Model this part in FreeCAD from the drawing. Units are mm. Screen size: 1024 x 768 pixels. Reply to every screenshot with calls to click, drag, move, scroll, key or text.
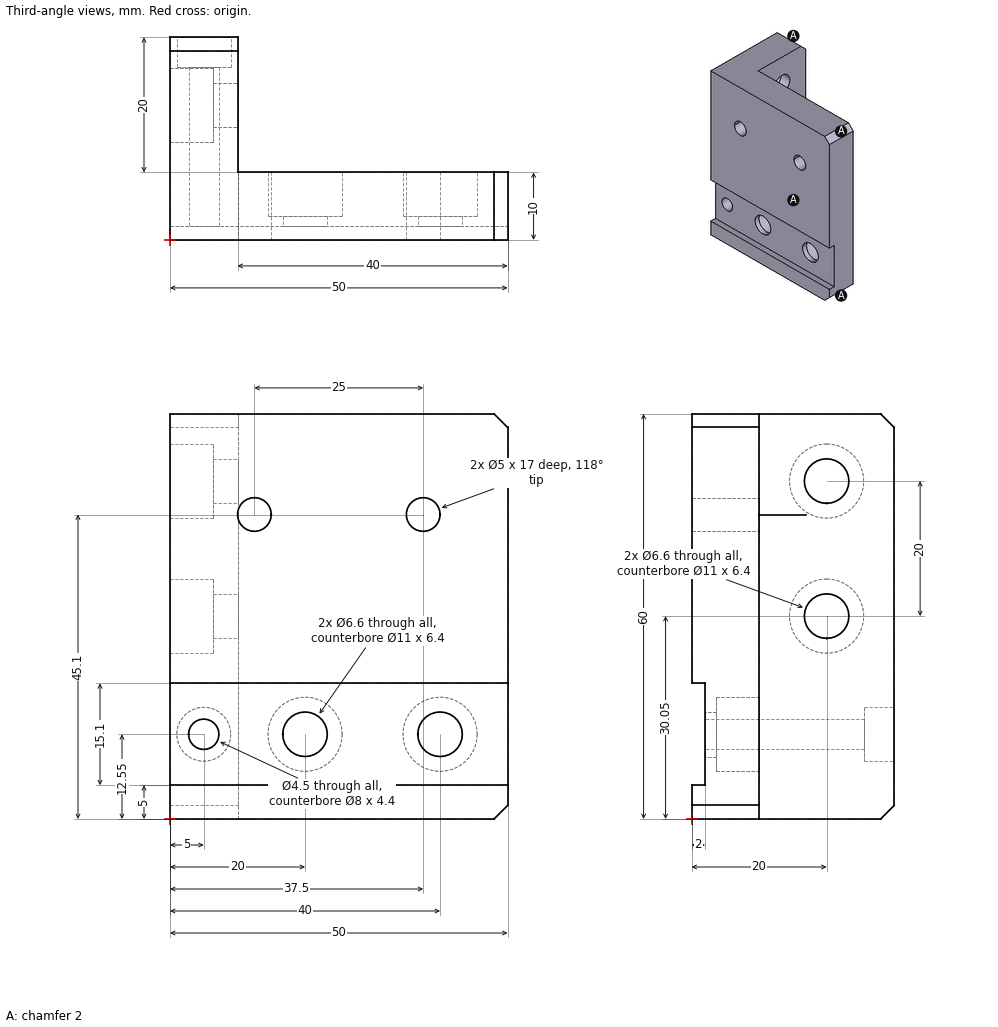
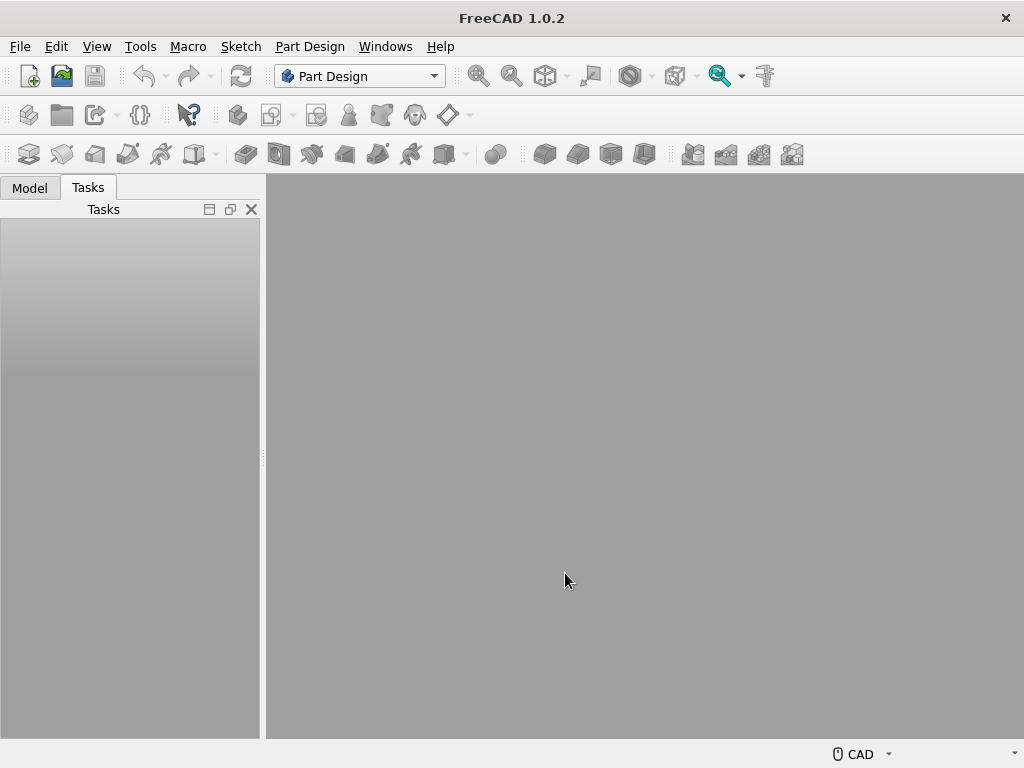
key(ctrl+n)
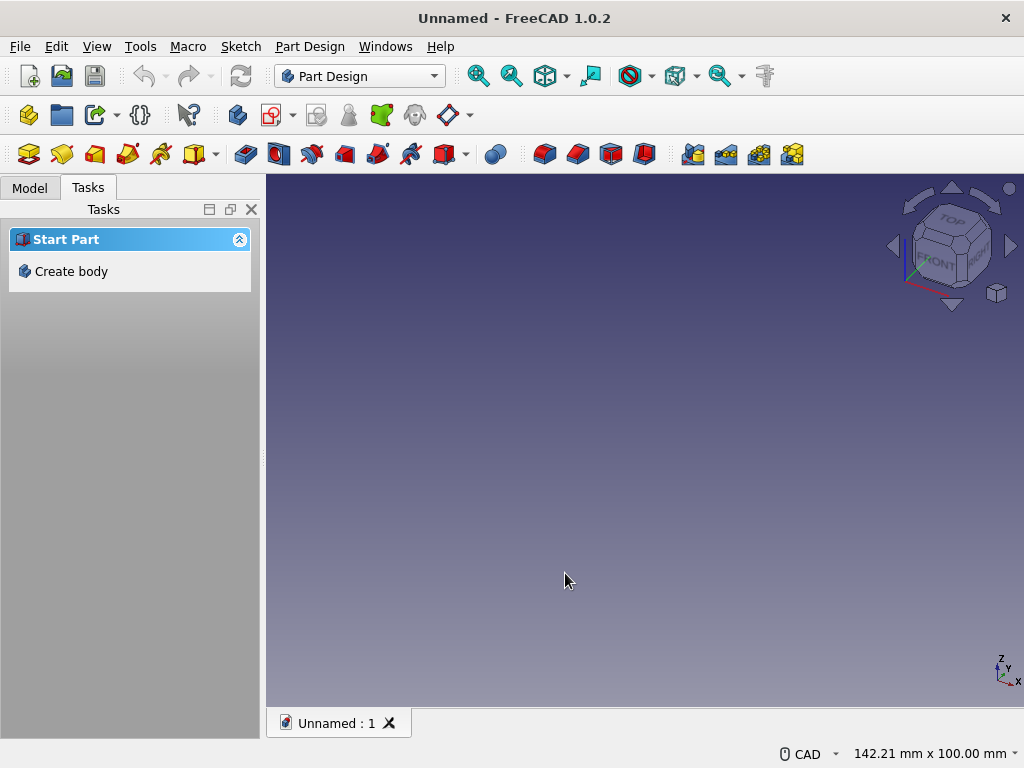
click(270, 116)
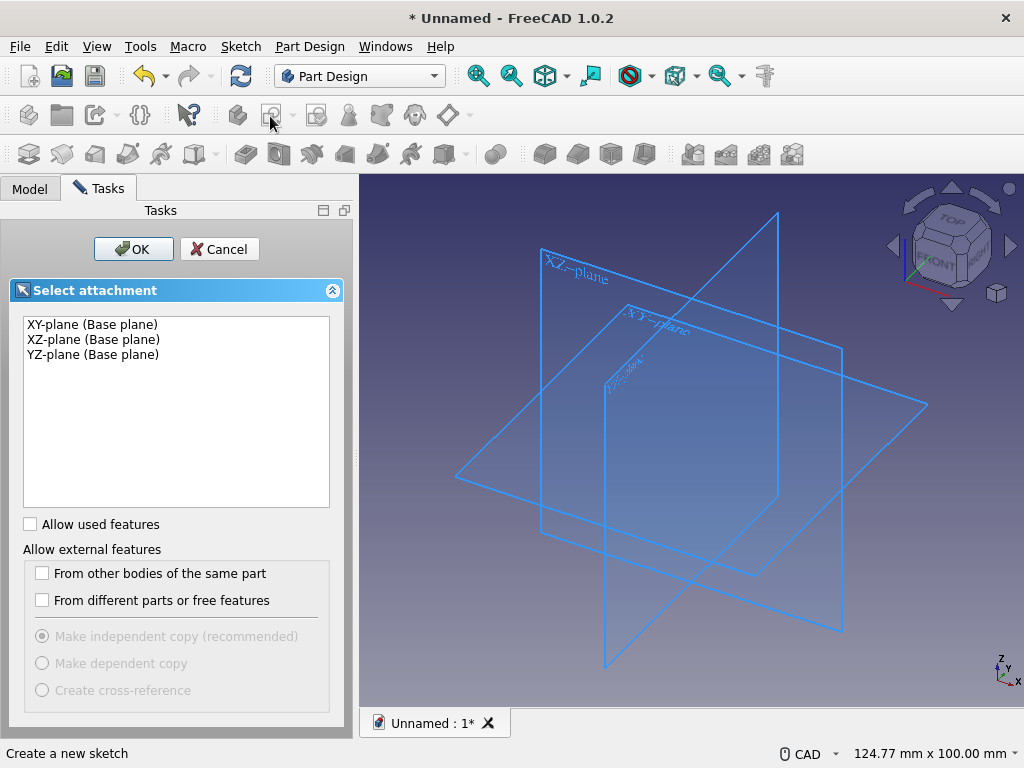
click(84, 324)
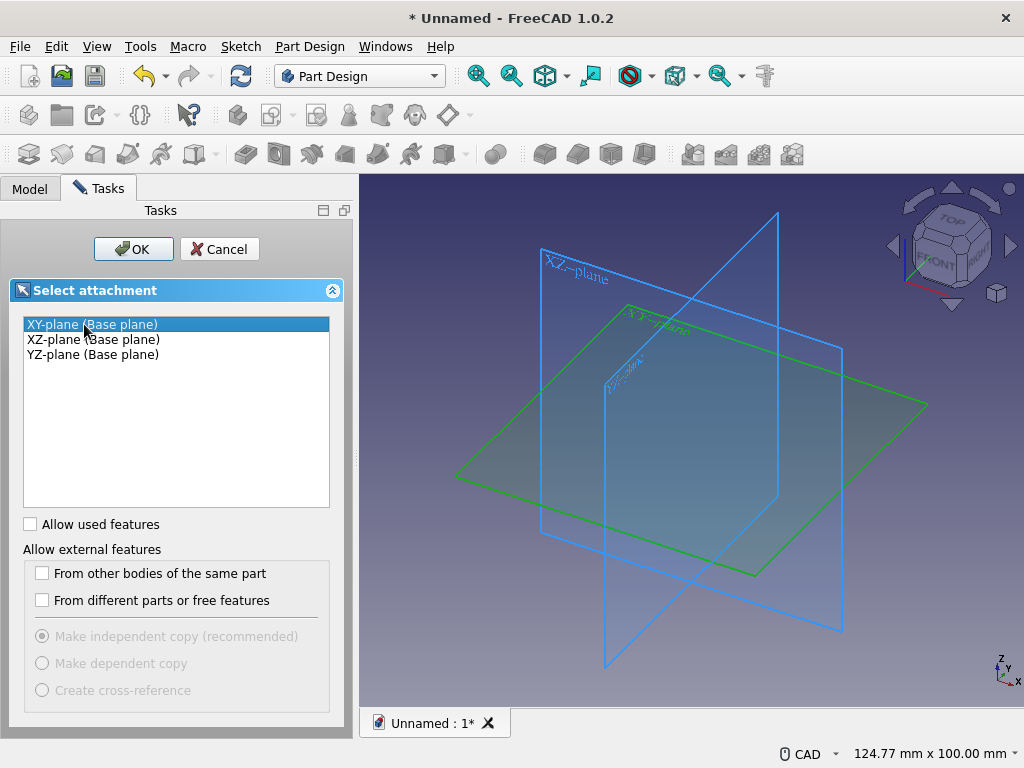
click(134, 249)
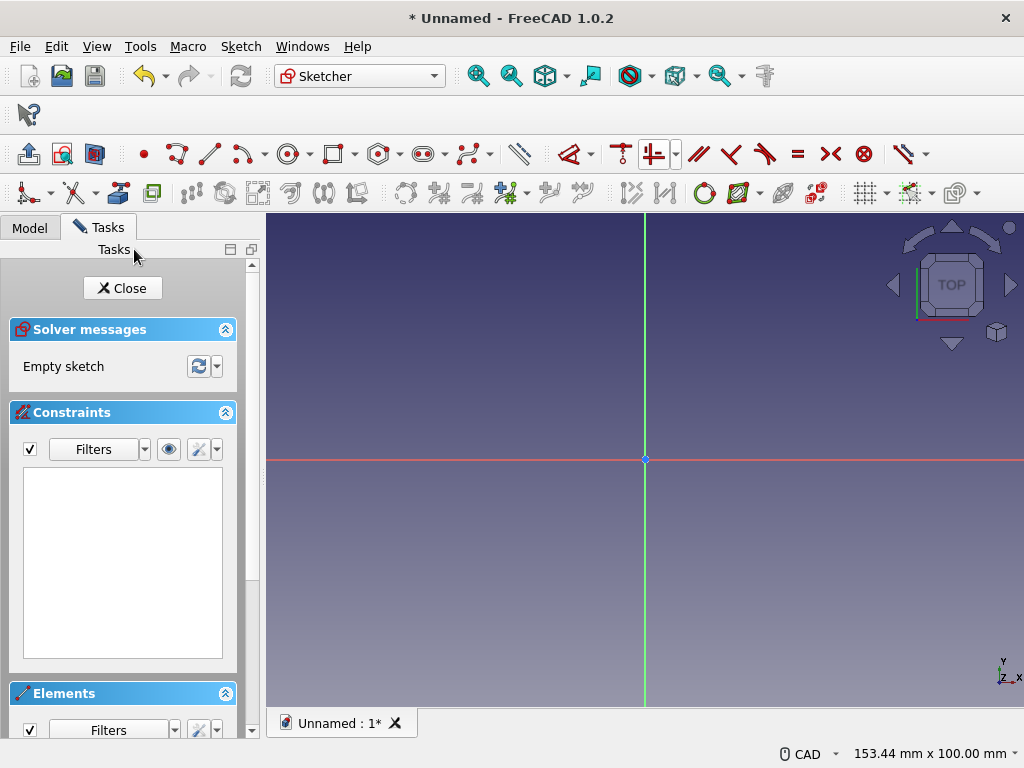
scroll(294, 679, down, 1)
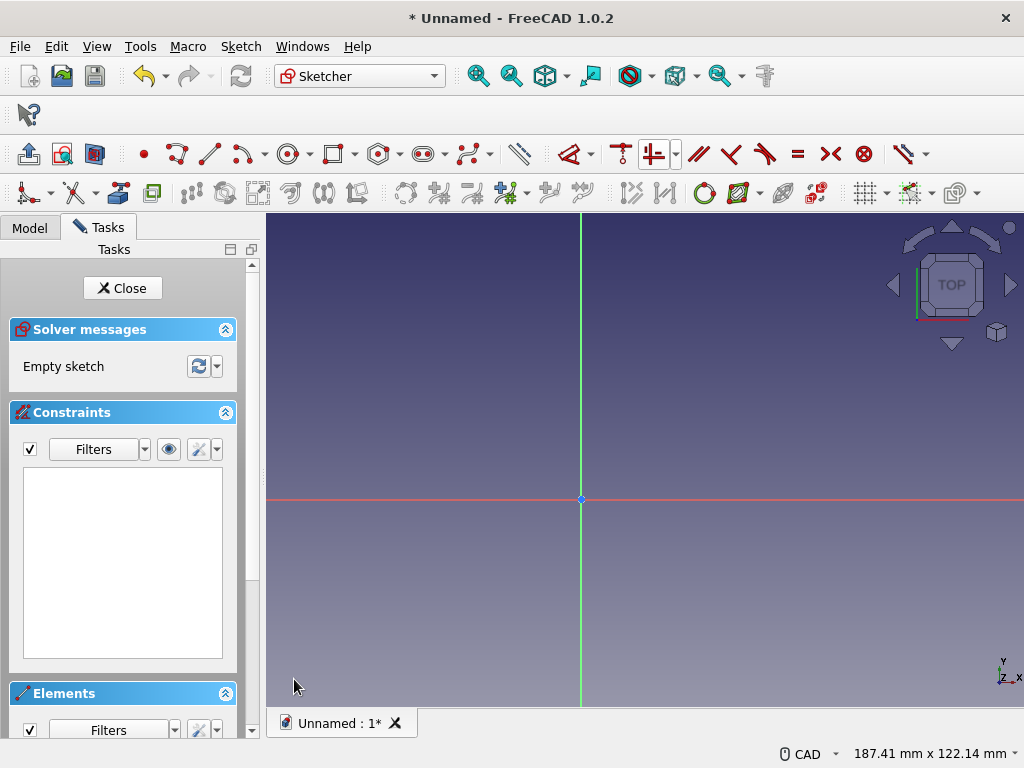
scroll(811, 414, up, 3)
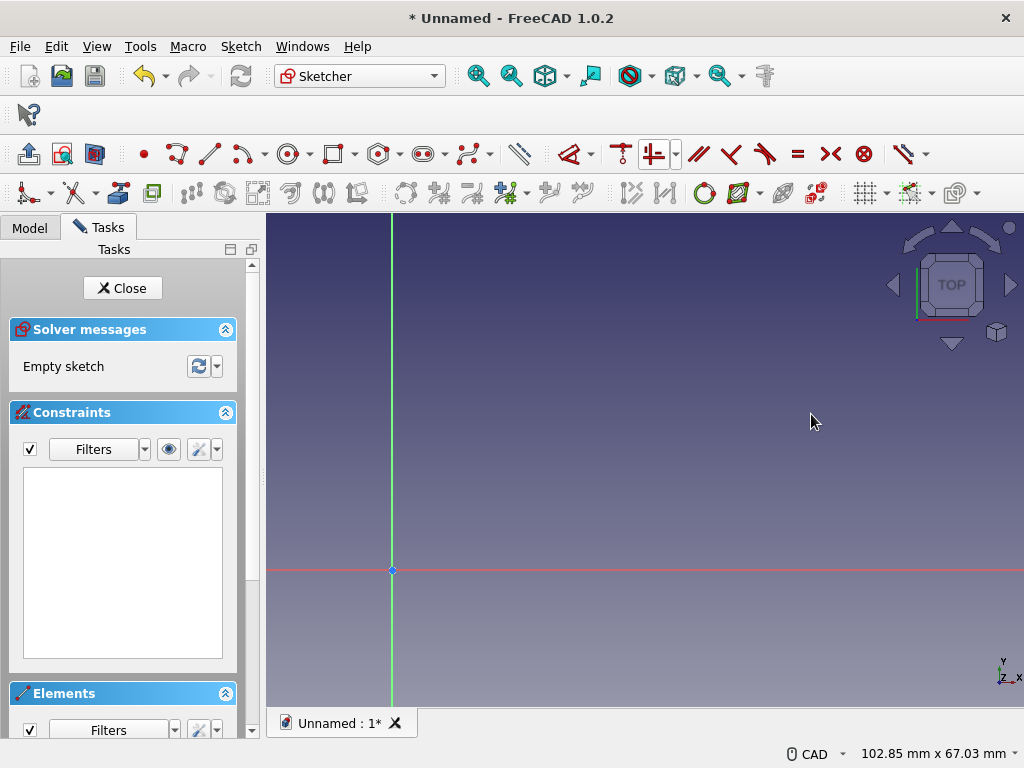
click(177, 154)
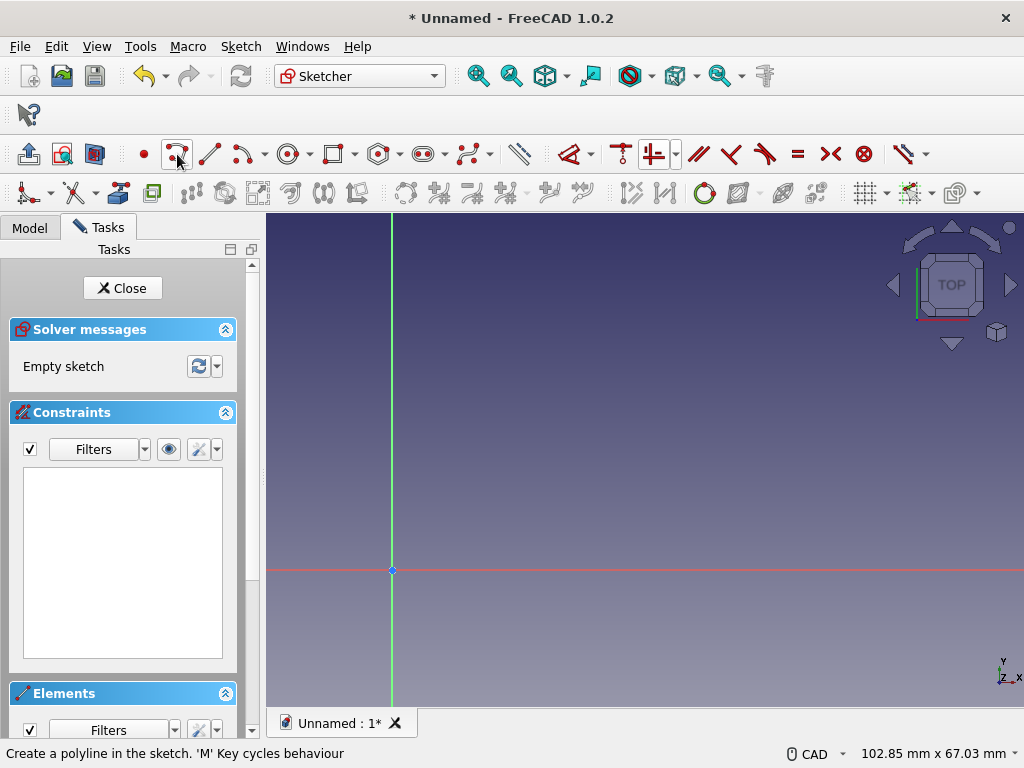
click(392, 570)
click(760, 561)
click(760, 496)
click(466, 496)
click(466, 349)
click(401, 349)
click(392, 570)
key(Escape)
key(Escape)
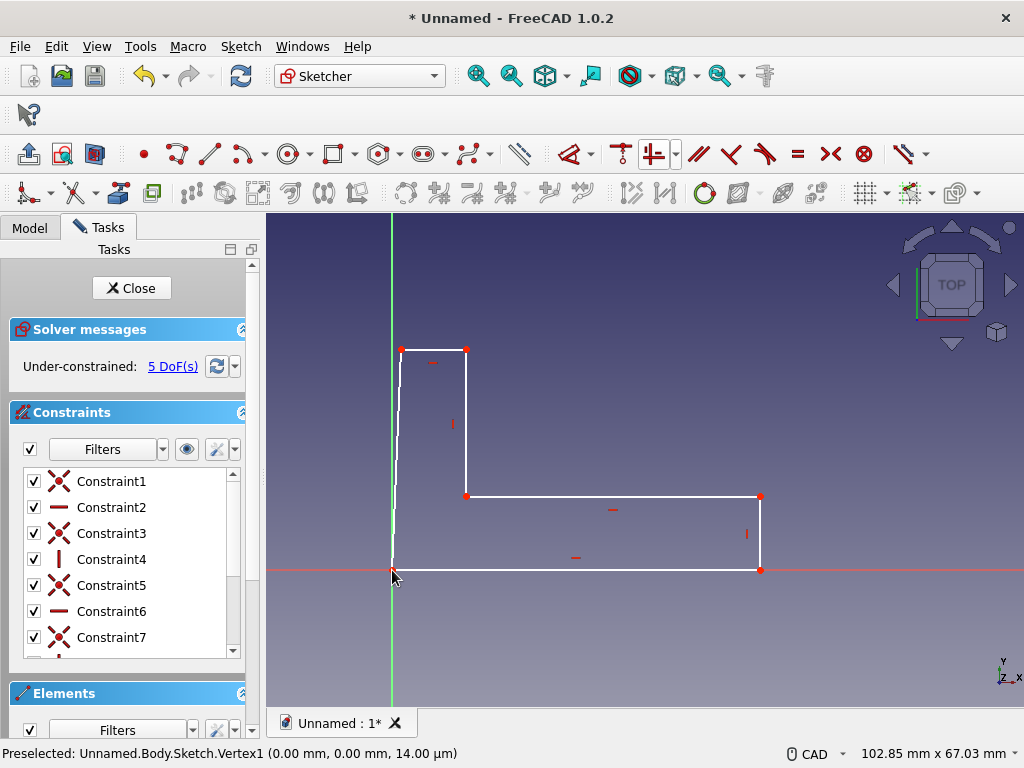
click(395, 504)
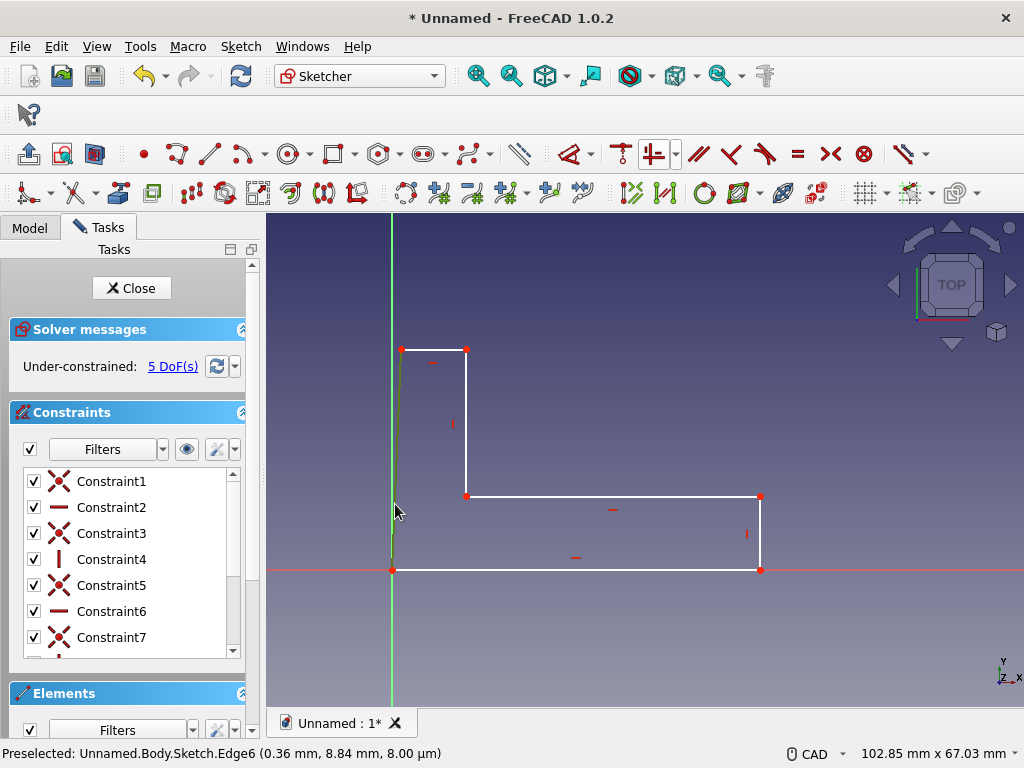
click(676, 154)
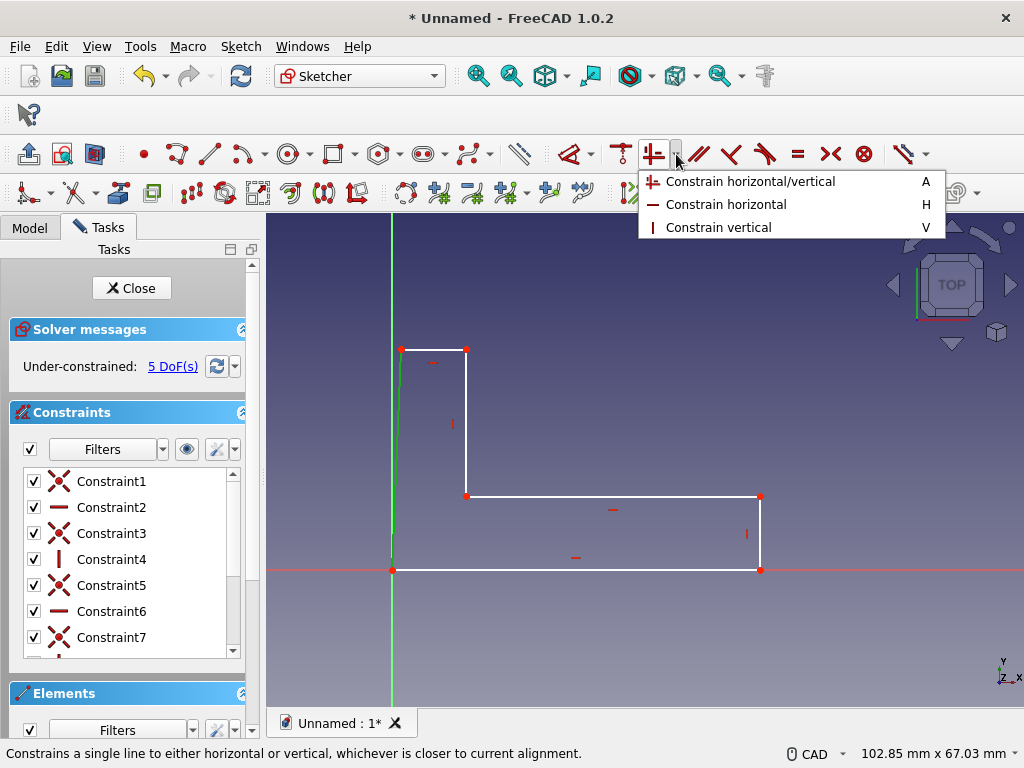
click(792, 228)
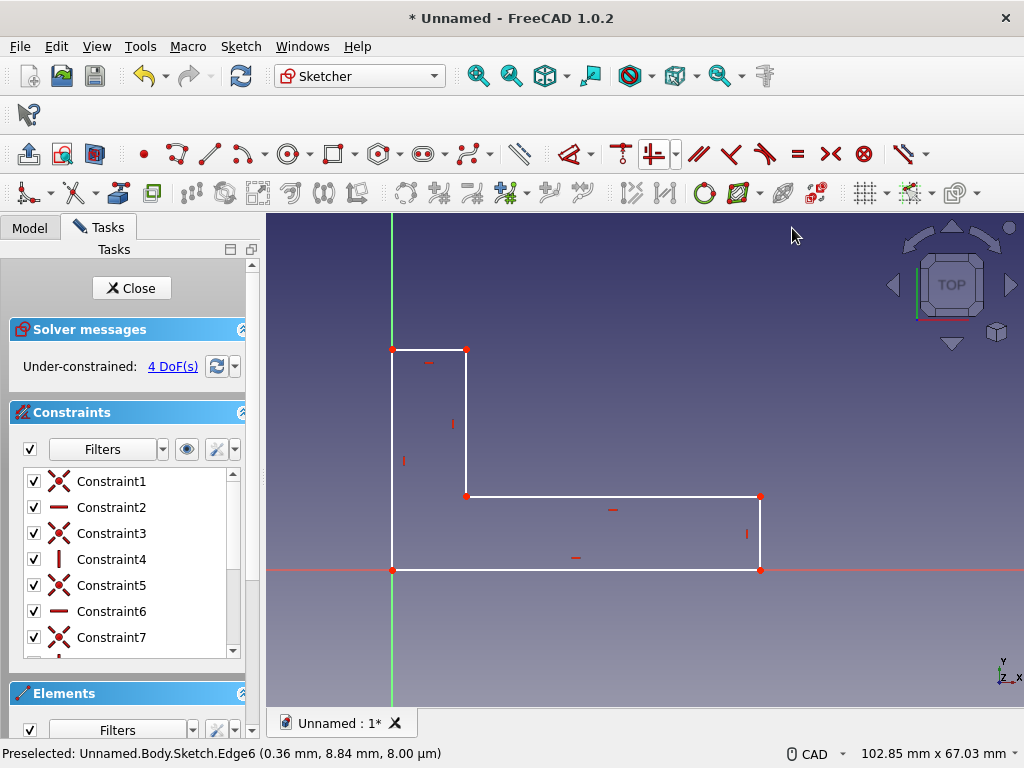
click(568, 154)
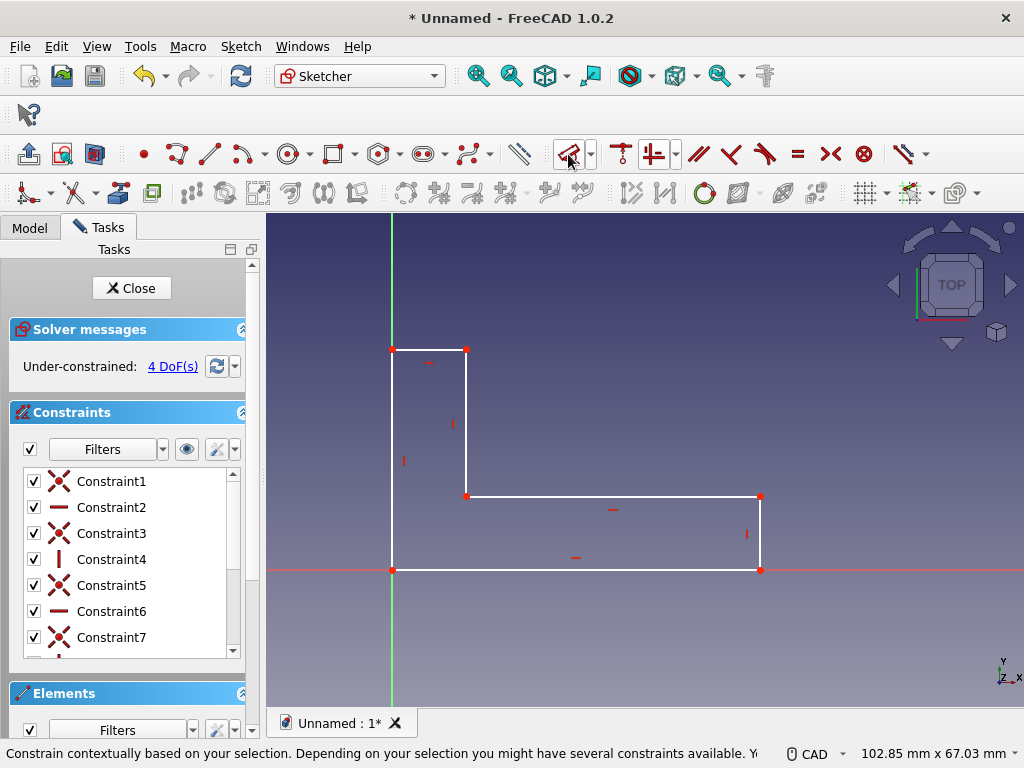
click(502, 570)
click(576, 604)